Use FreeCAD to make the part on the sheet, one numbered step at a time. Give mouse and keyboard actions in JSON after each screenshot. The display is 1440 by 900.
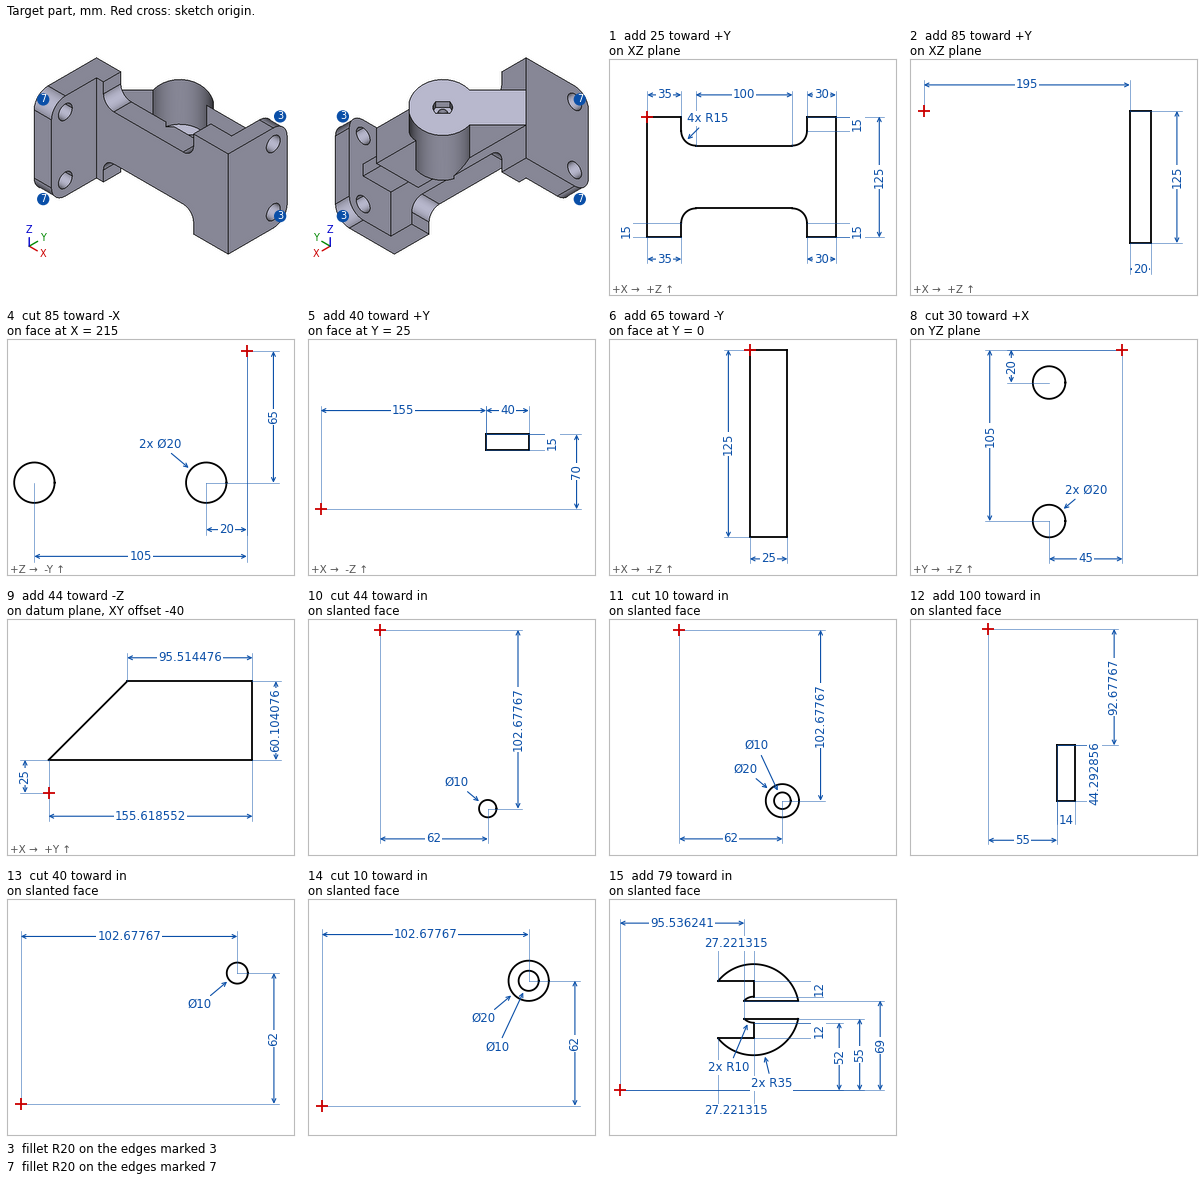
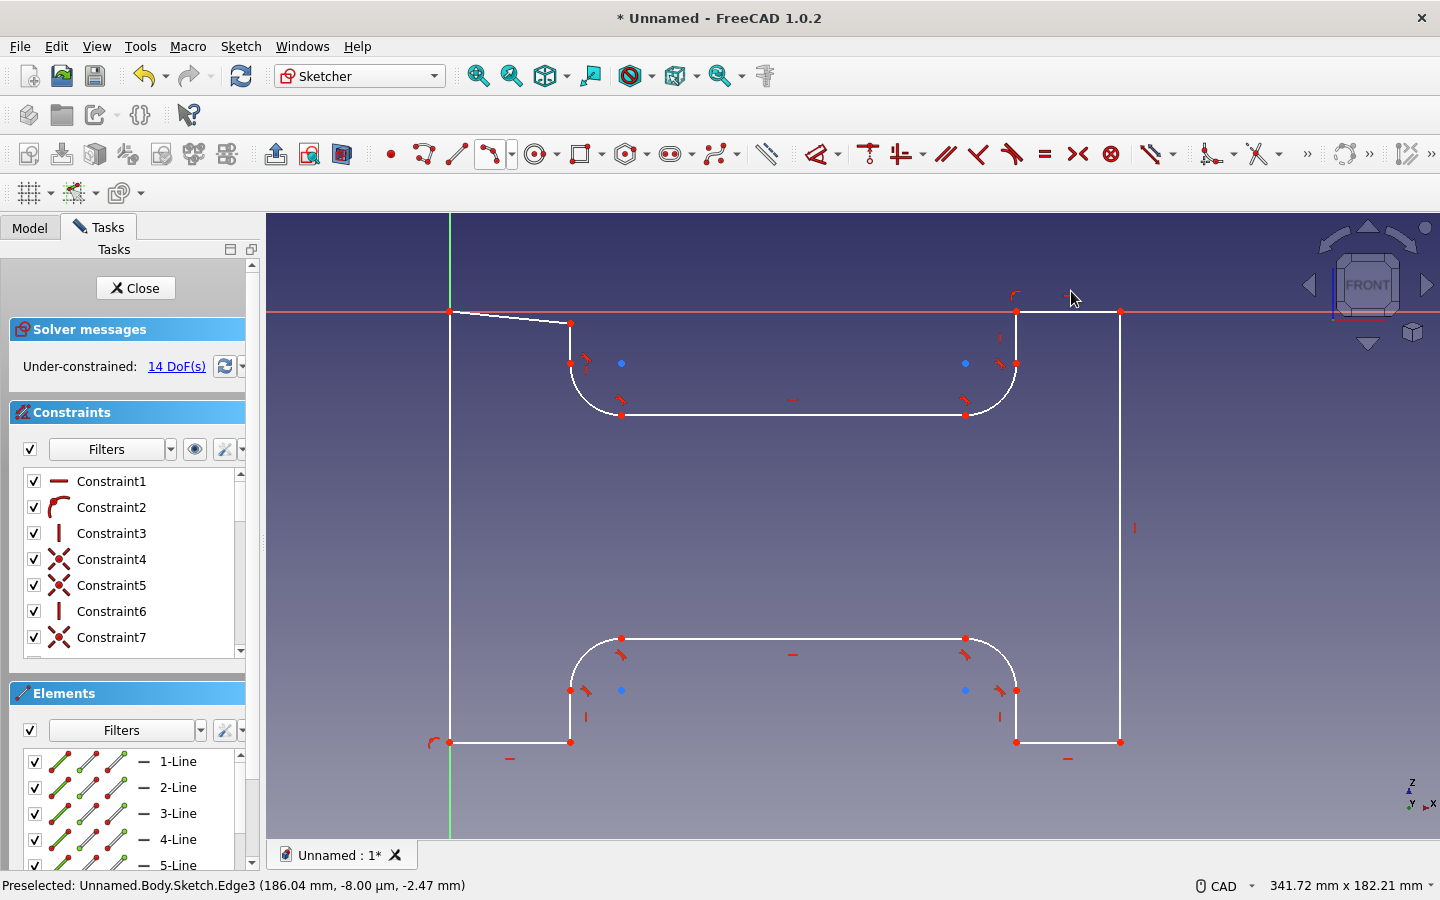
{"action": "scroll", "coordinate": [534, 320], "scroll_direction": "up", "scroll_amount": 3}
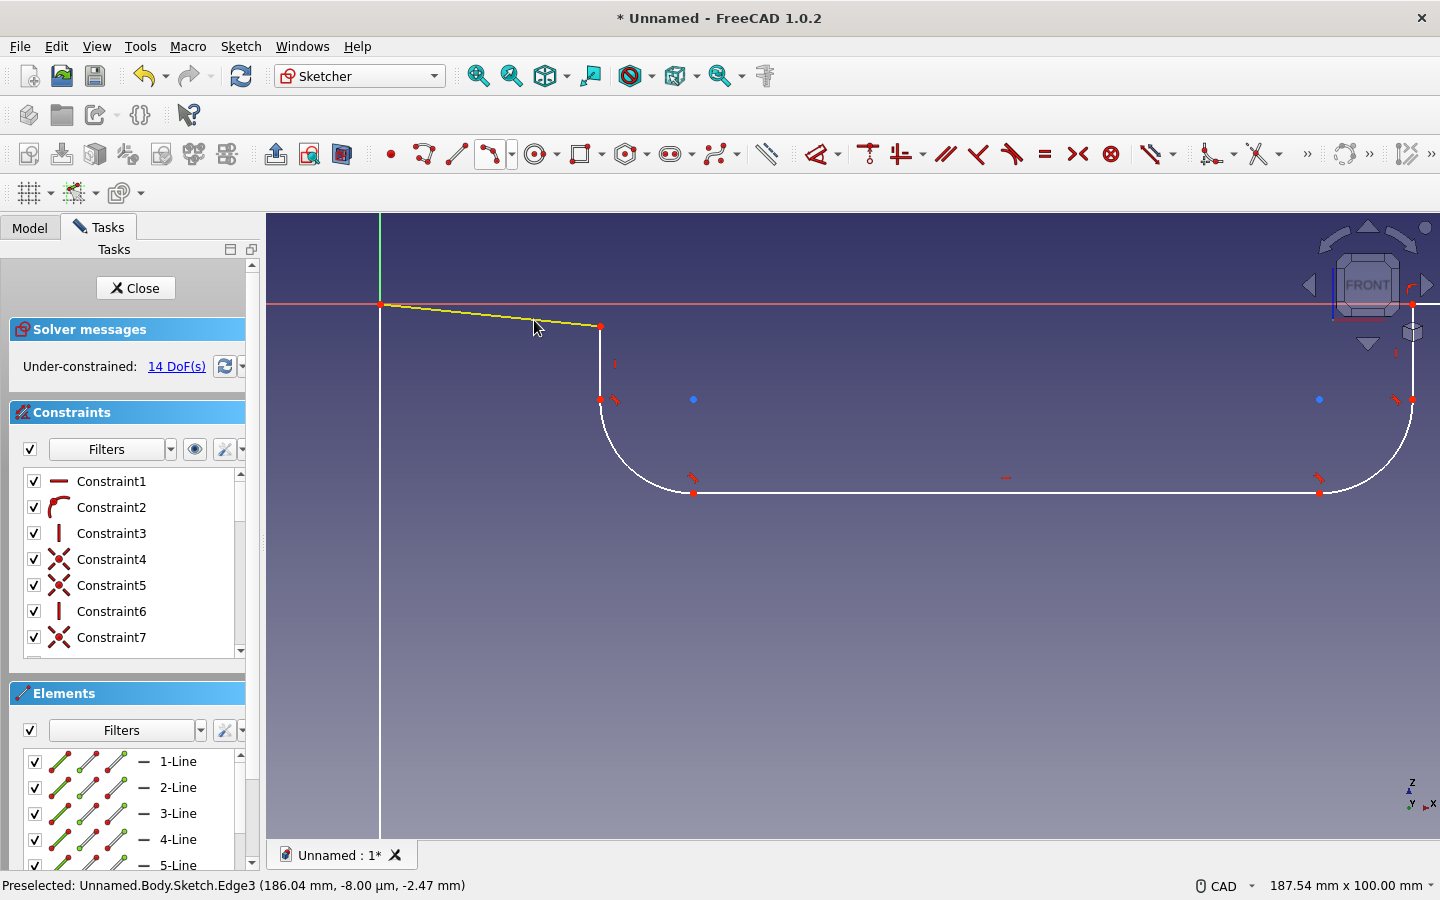
{"action": "left_click", "coordinate": [534, 320]}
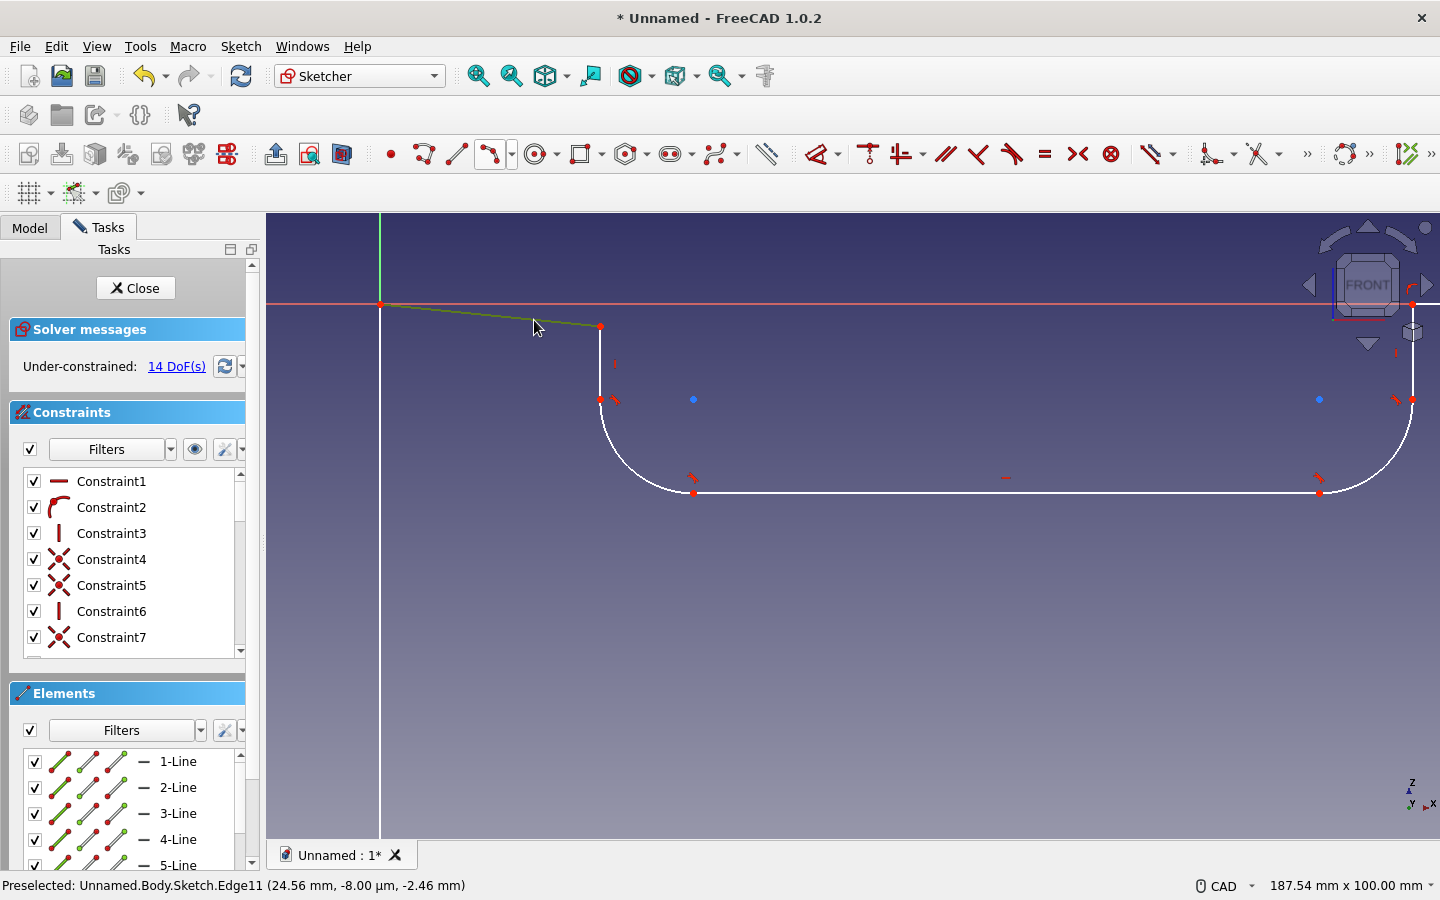
{"action": "key", "text": "h"}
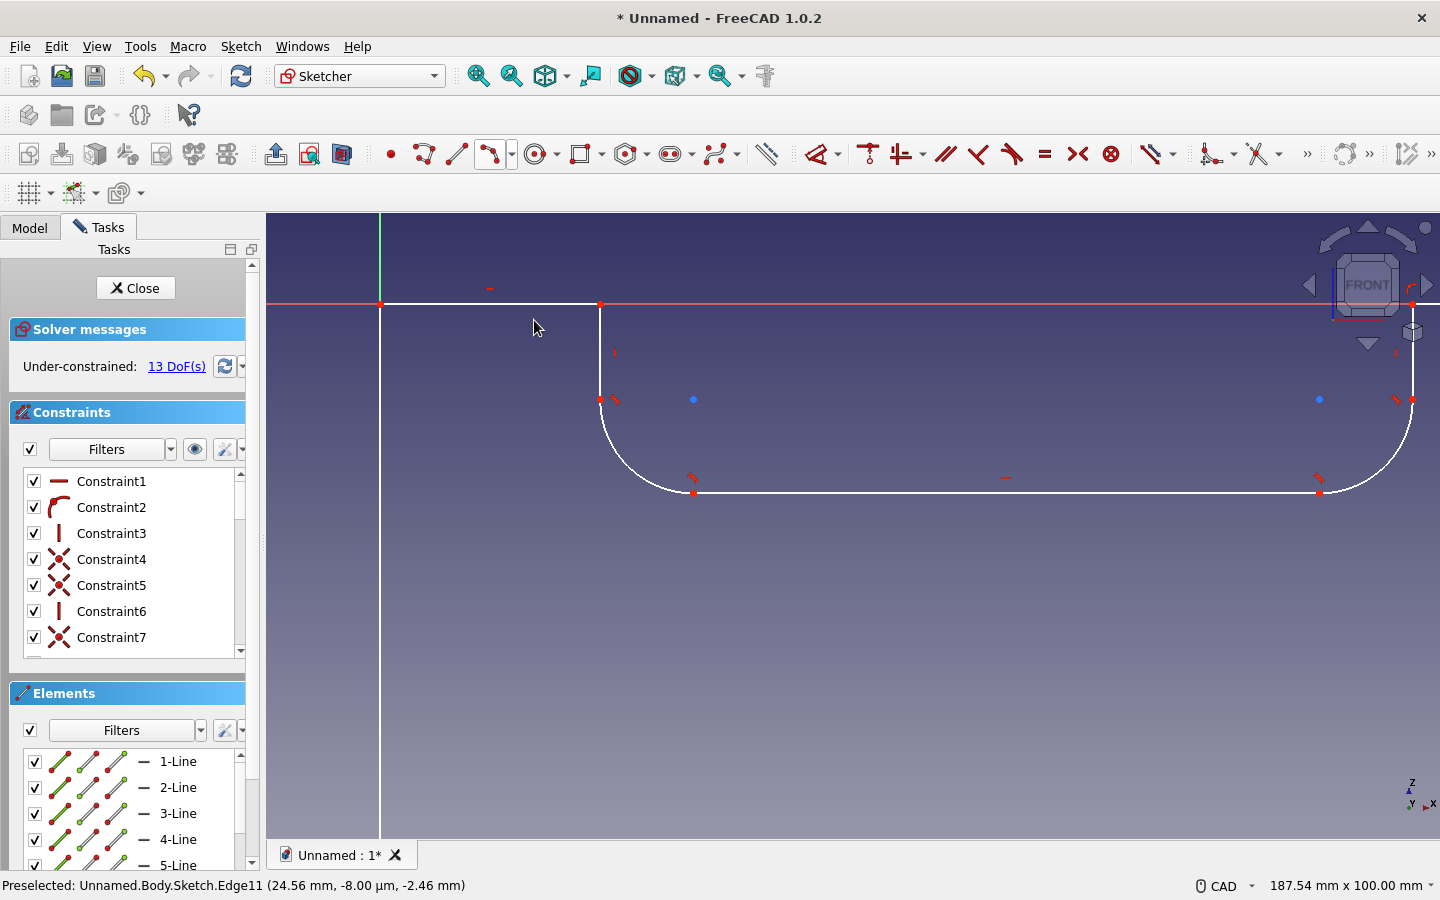
{"action": "scroll", "coordinate": [534, 320], "scroll_direction": "down", "scroll_amount": 3}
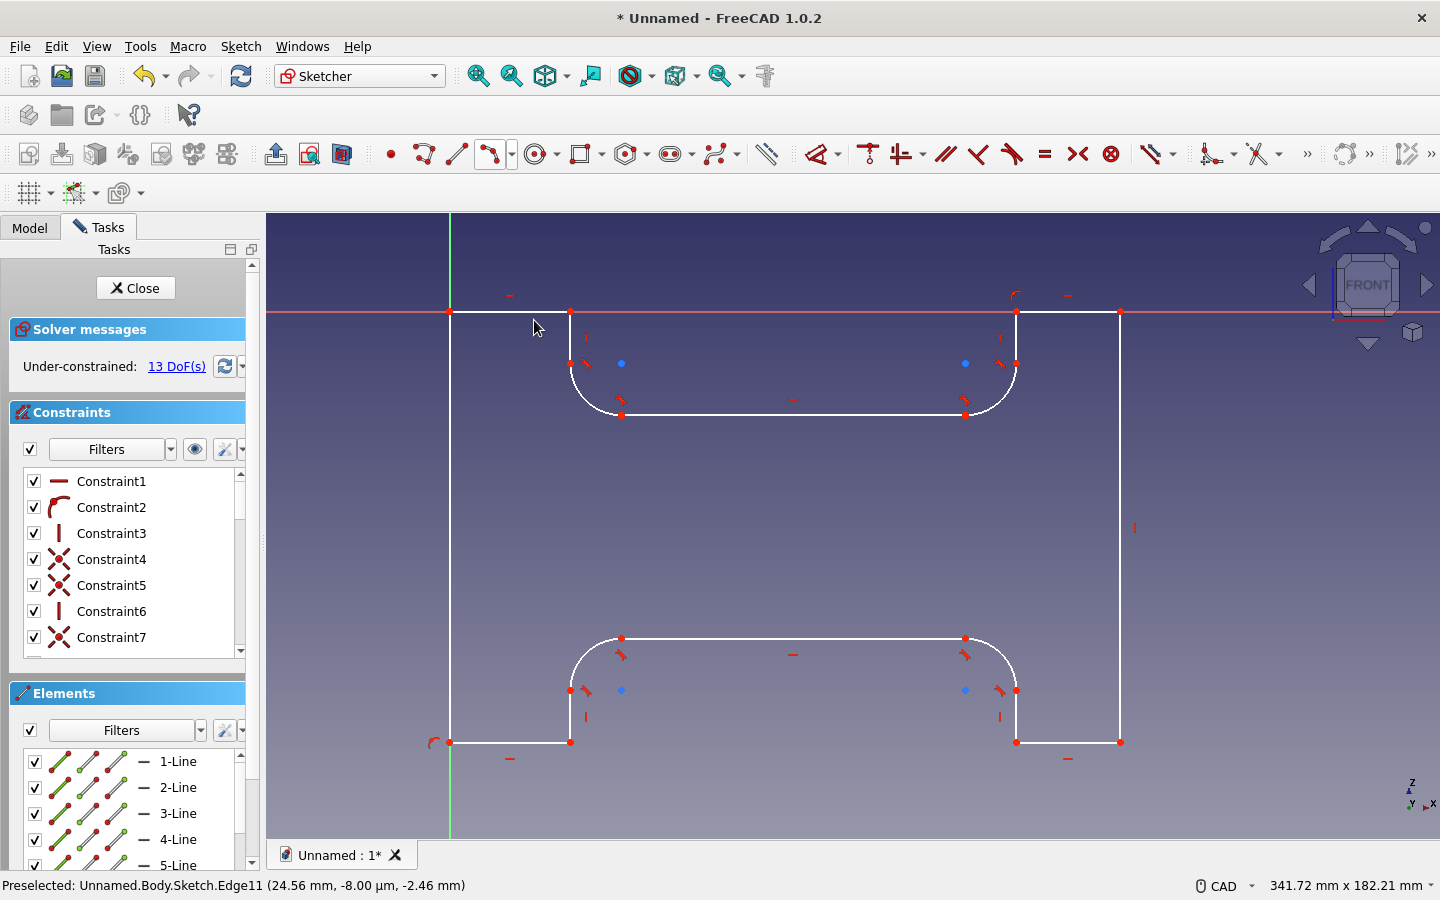
{"action": "left_click", "coordinate": [988, 410]}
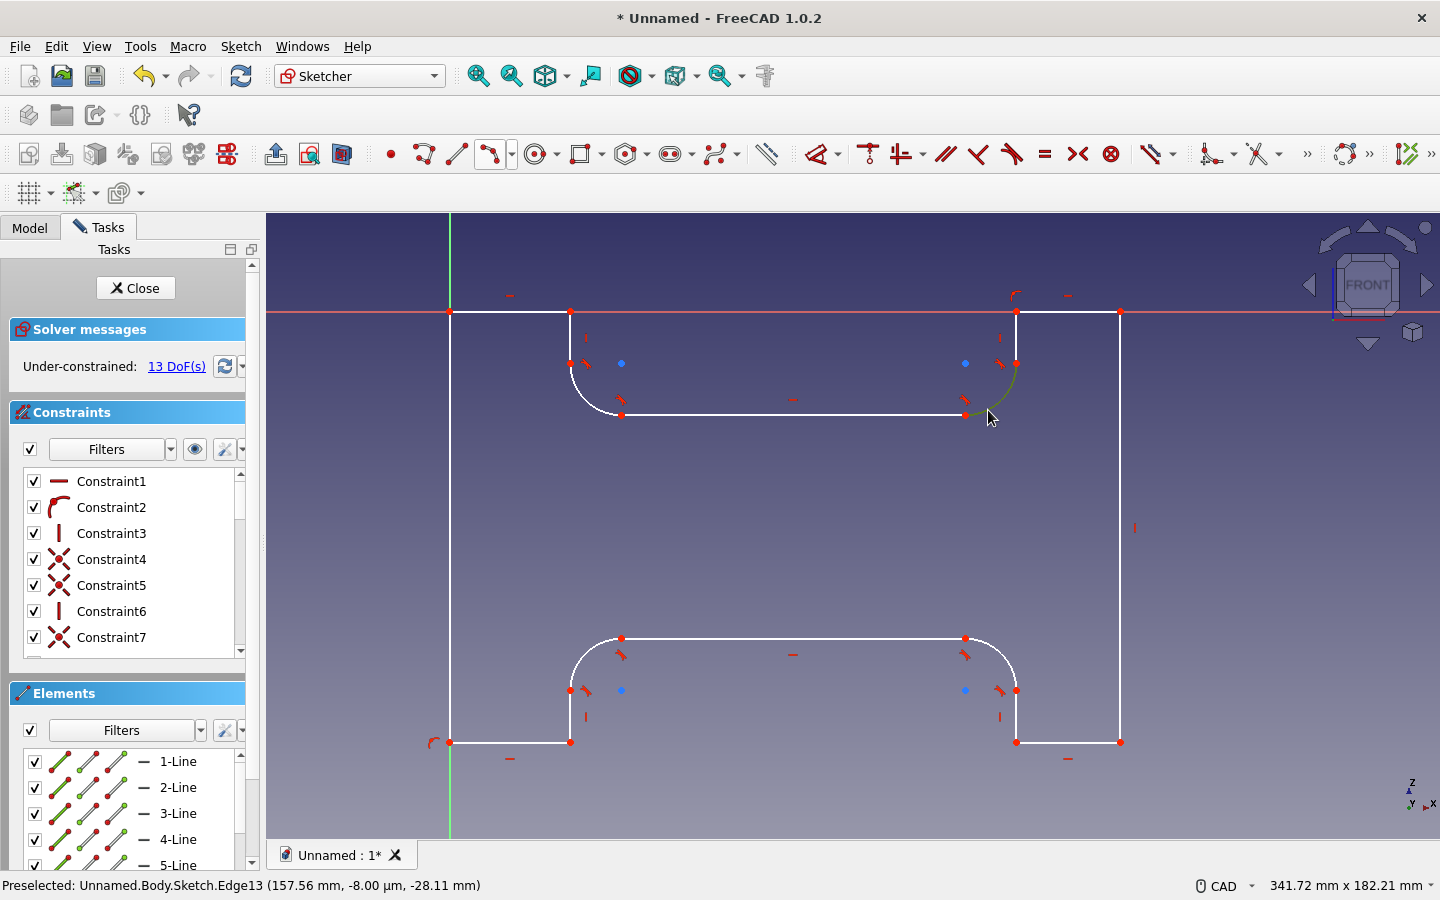
{"action": "left_click", "coordinate": [1011, 667]}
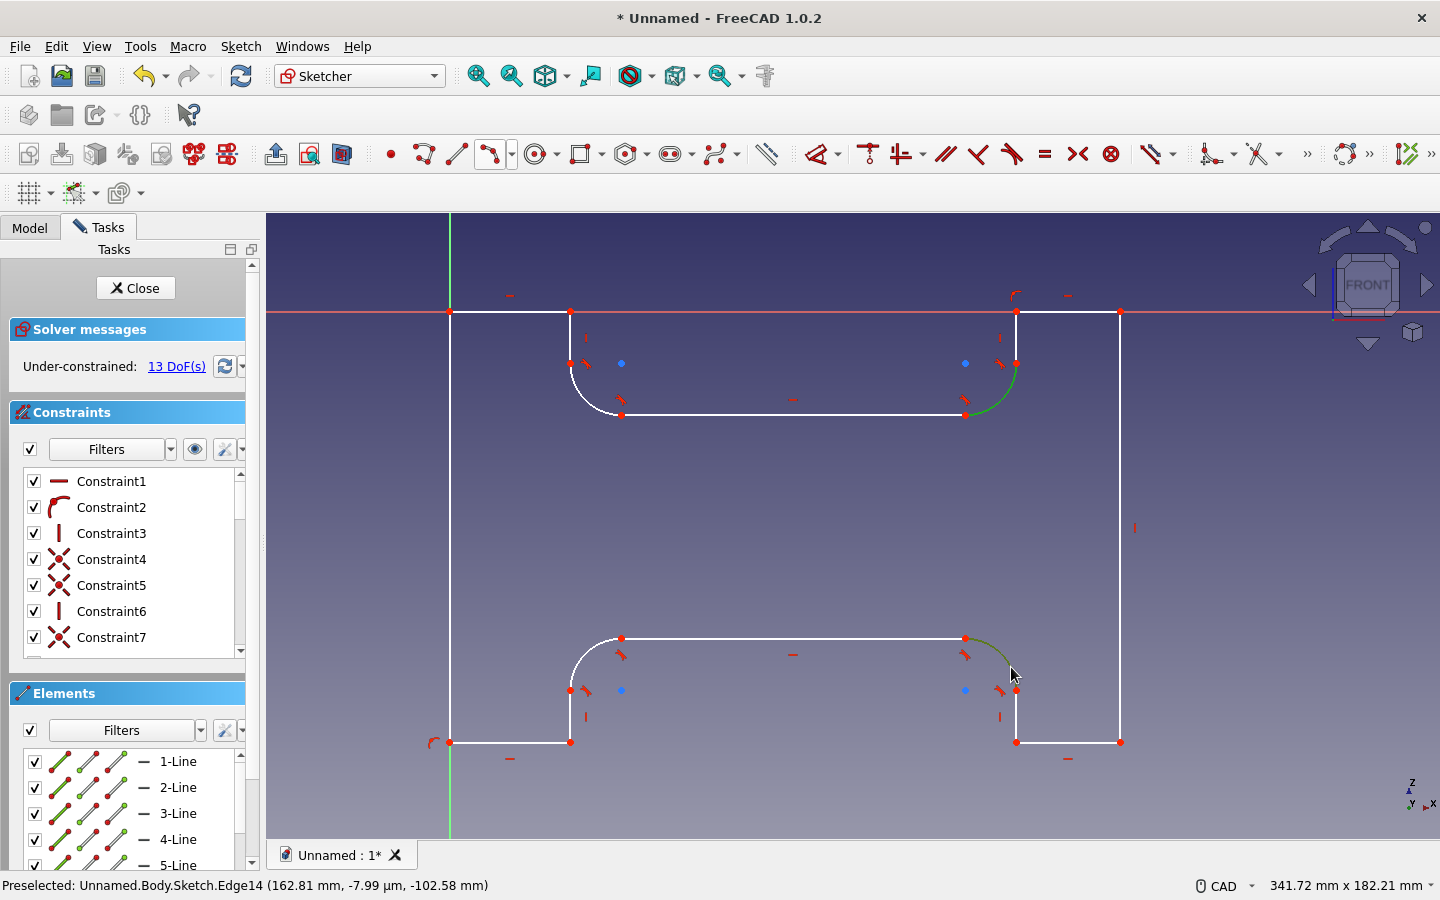
{"action": "left_click", "coordinate": [598, 644]}